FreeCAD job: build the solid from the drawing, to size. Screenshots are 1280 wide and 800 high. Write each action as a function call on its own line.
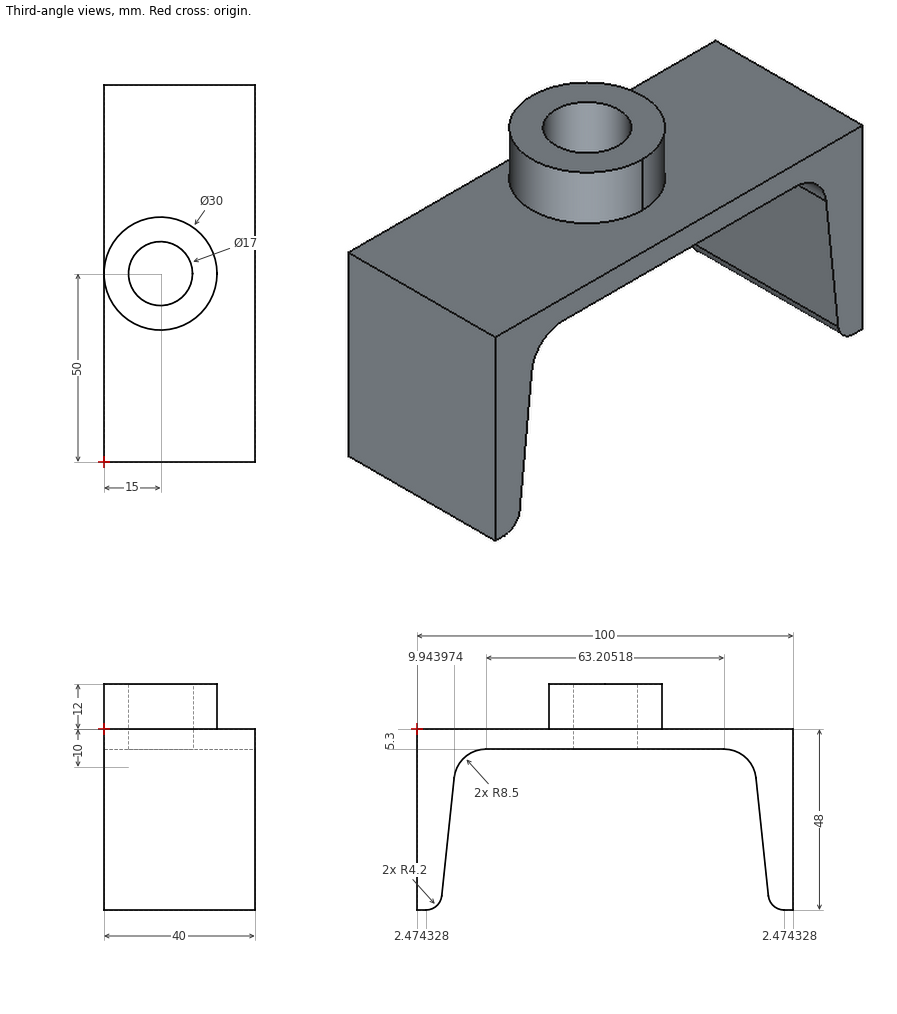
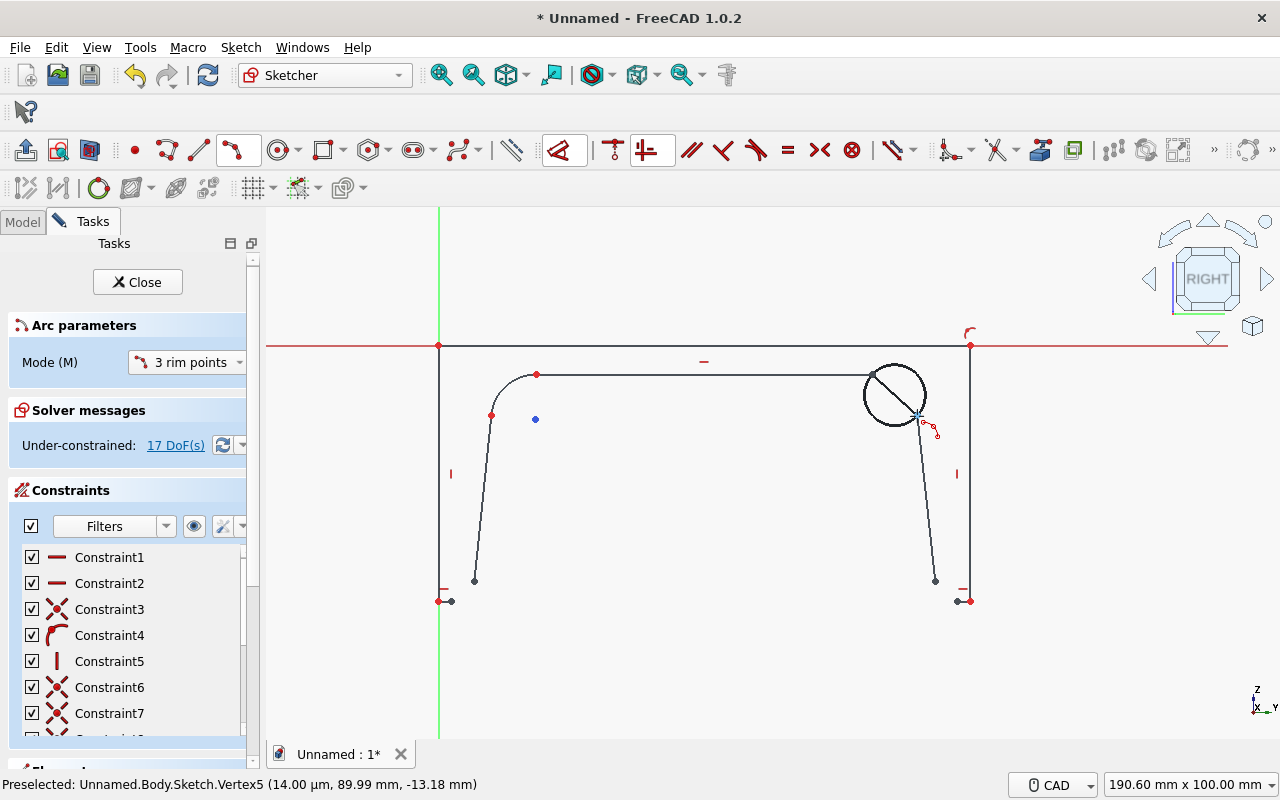
scroll(903, 385, up, 2)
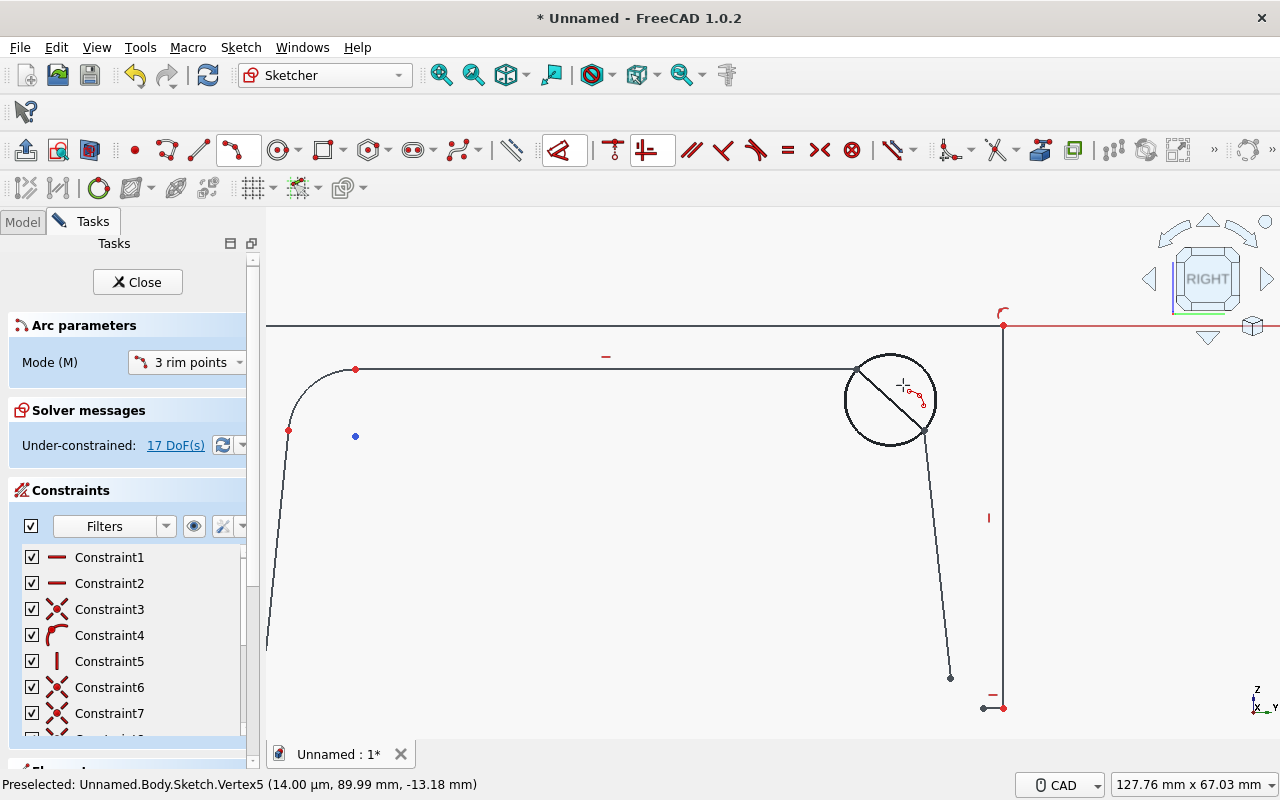
click(903, 385)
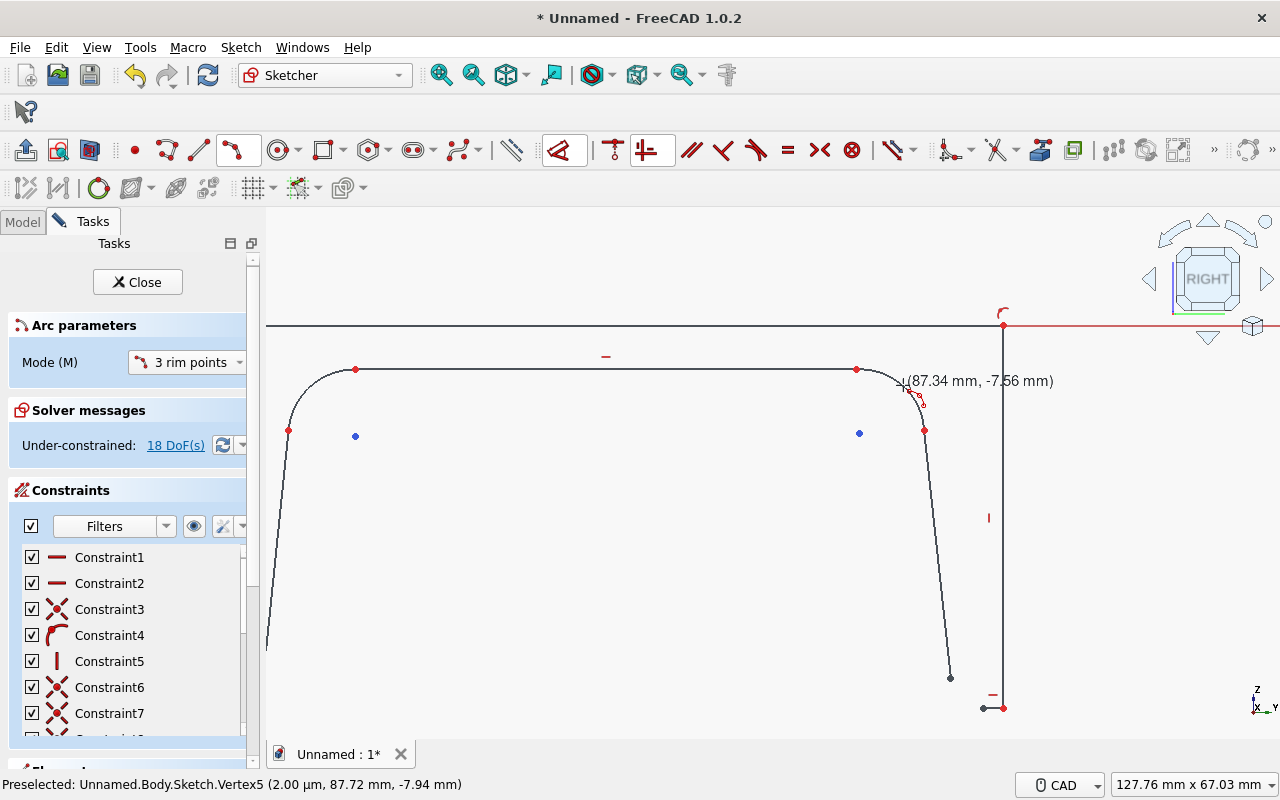
click(951, 678)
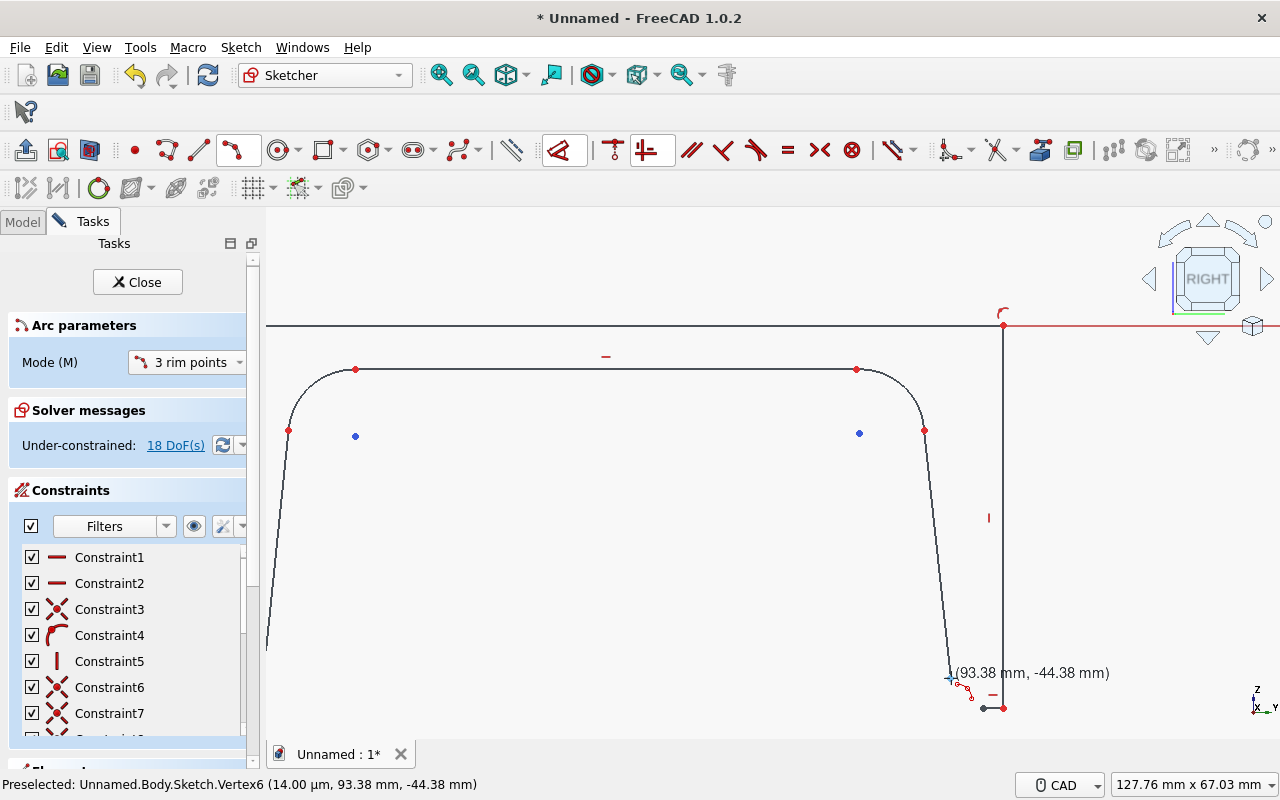
scroll(984, 707, up, 3)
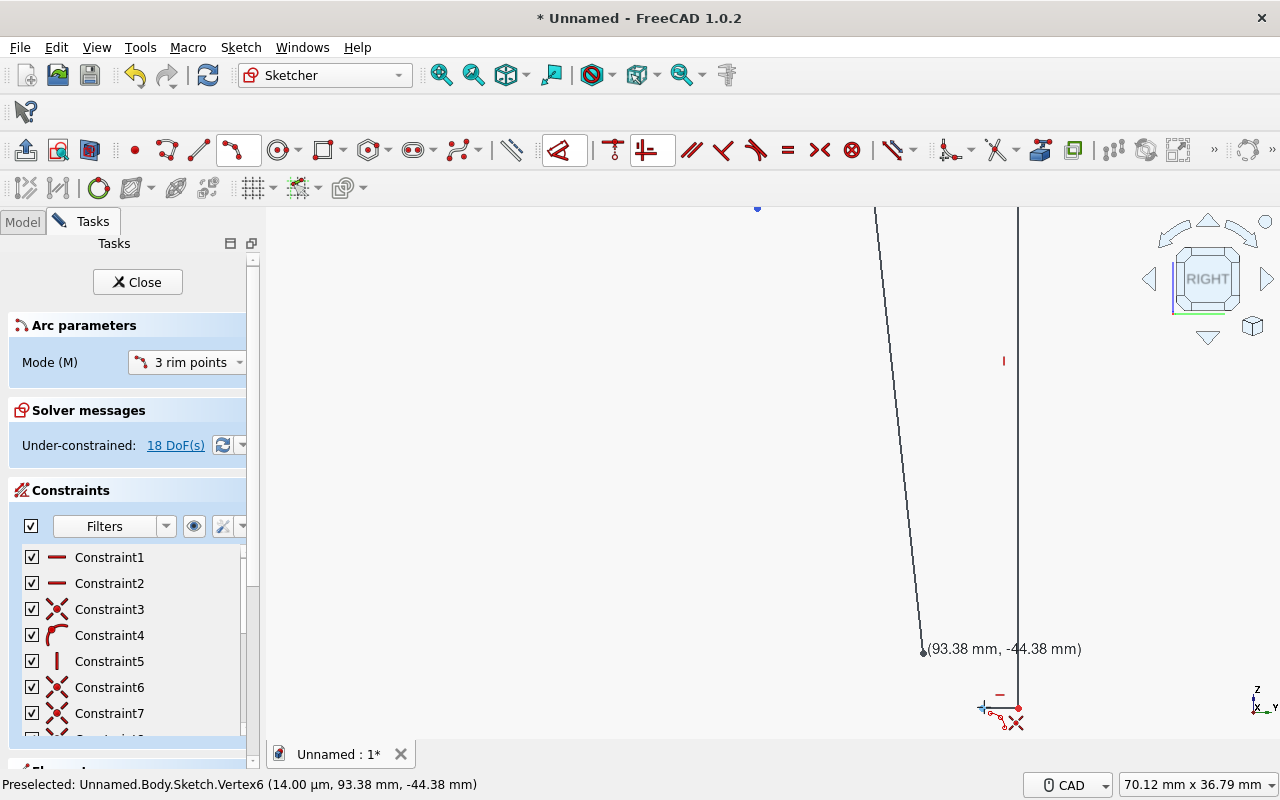
click(983, 708)
click(942, 690)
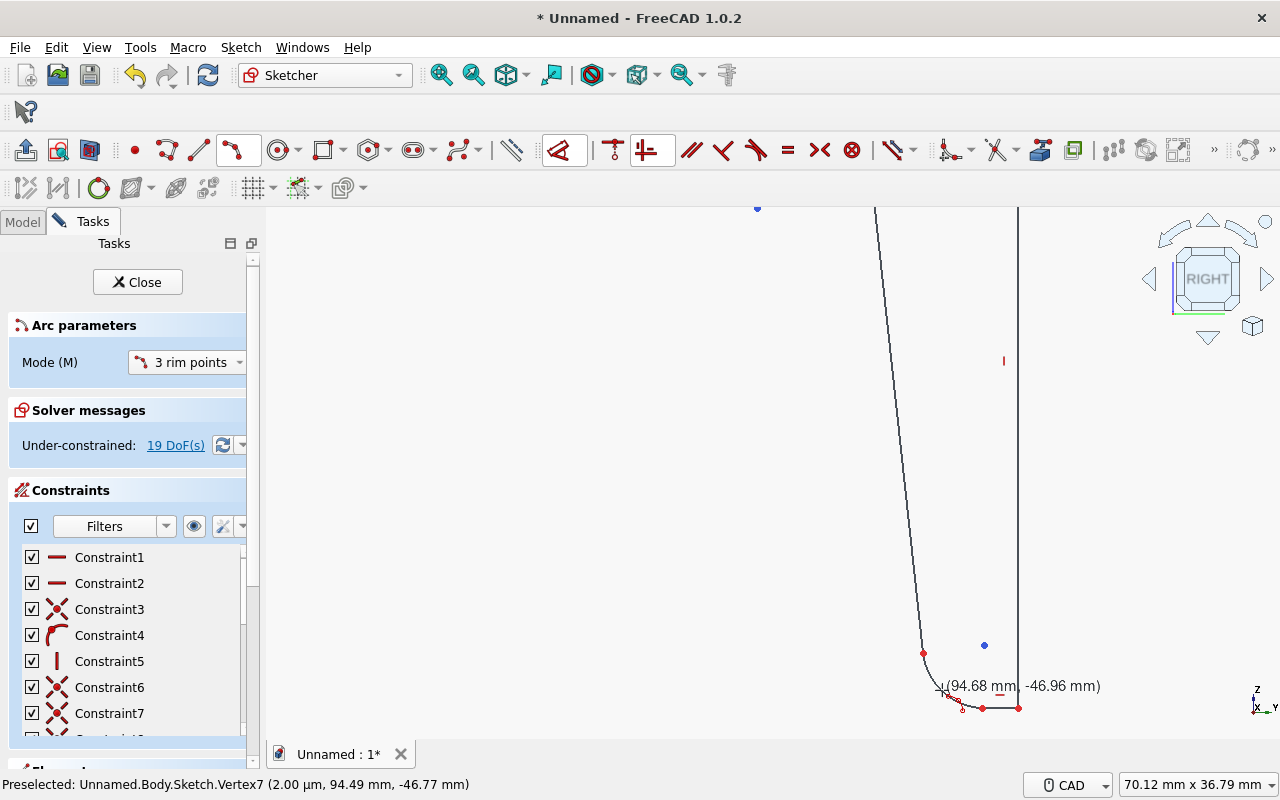
scroll(942, 539, down, 5)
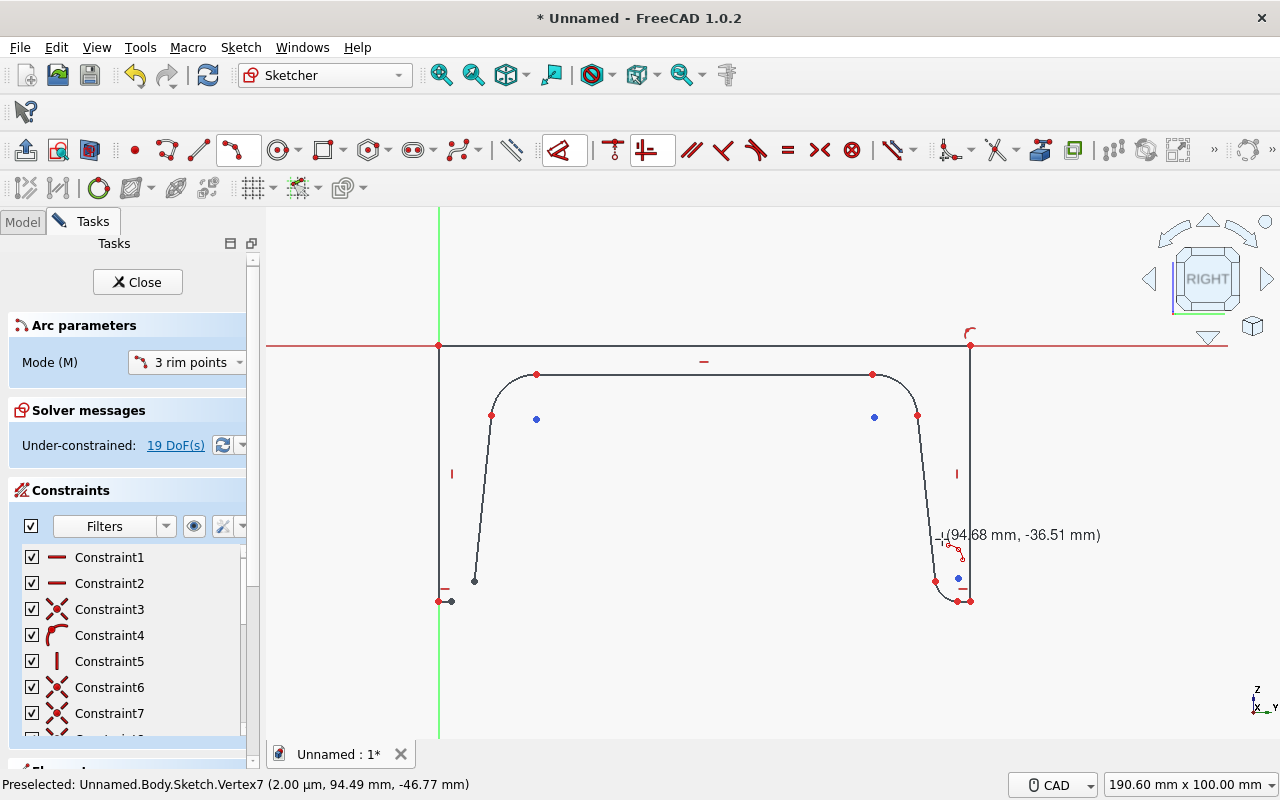
scroll(452, 601, up, 5)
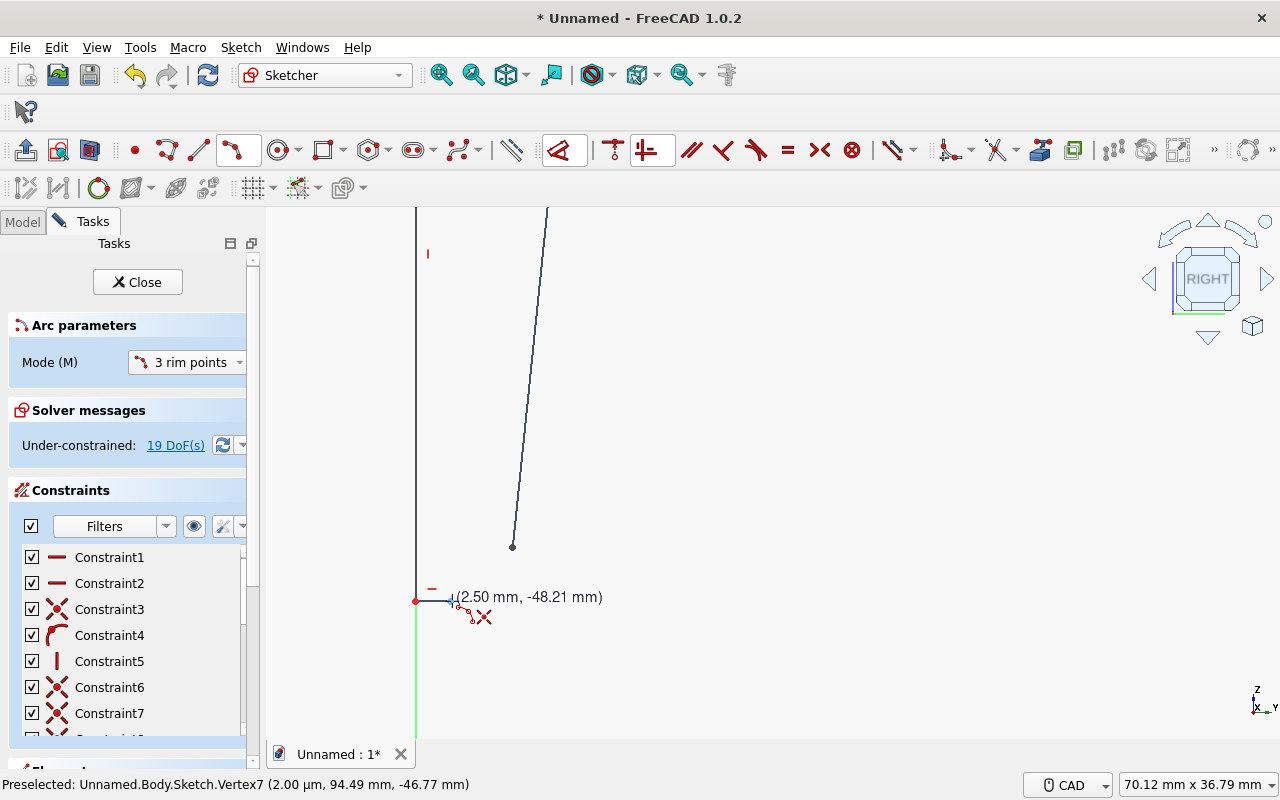
click(450, 601)
click(513, 547)
click(492, 584)
key(Escape)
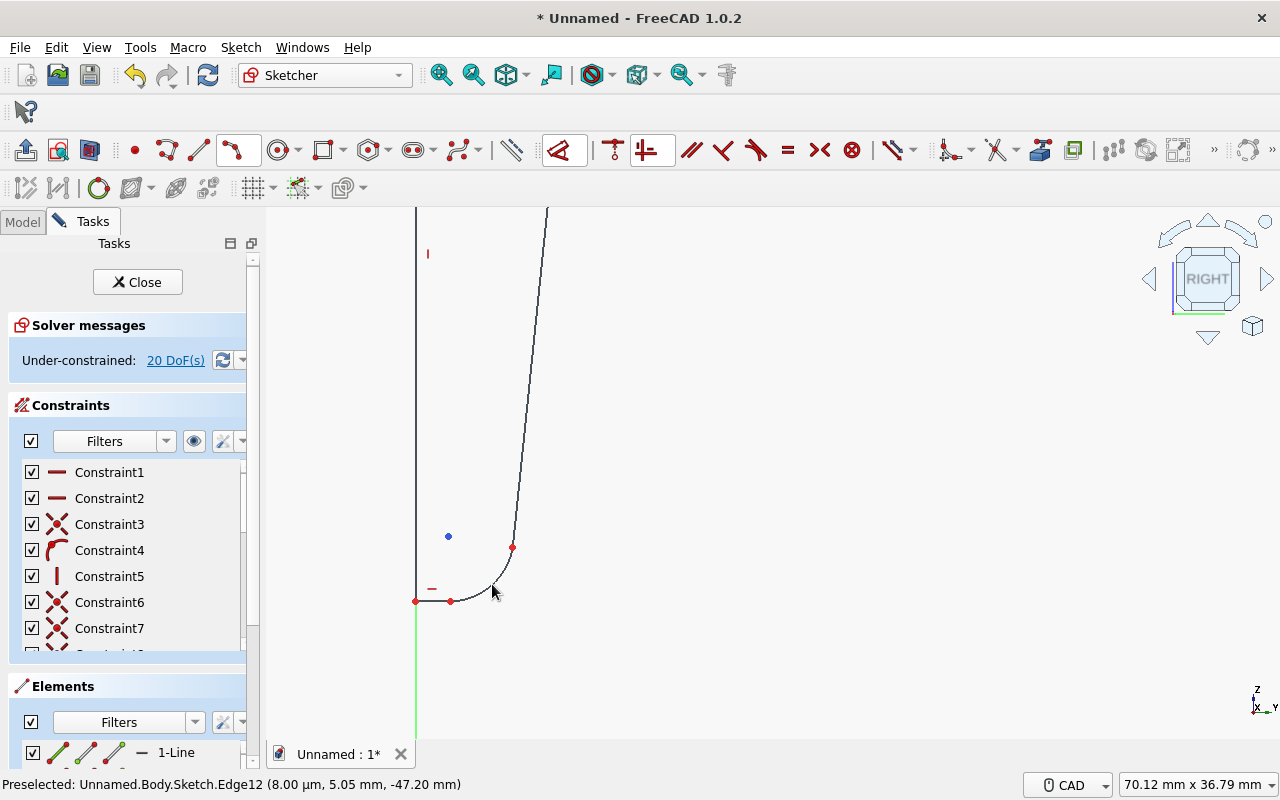
click(527, 412)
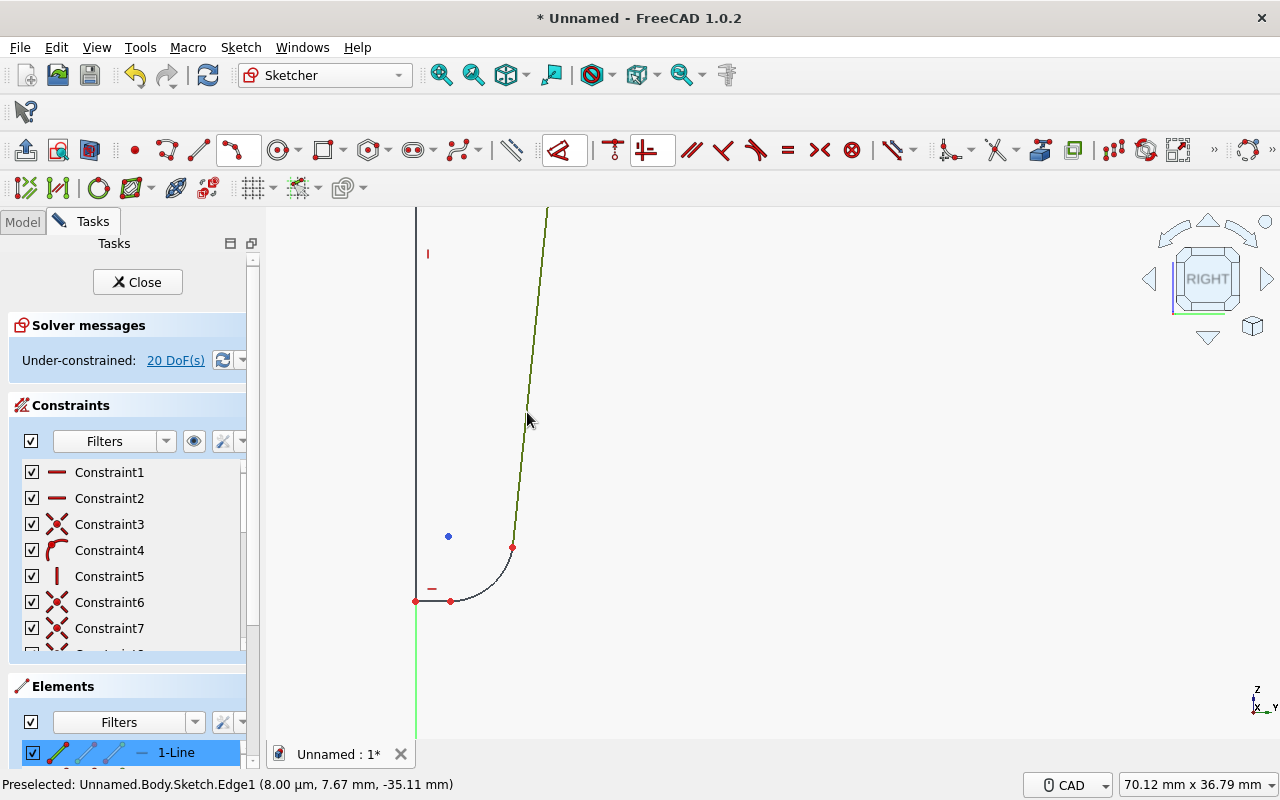
scroll(452, 601, down, 5)